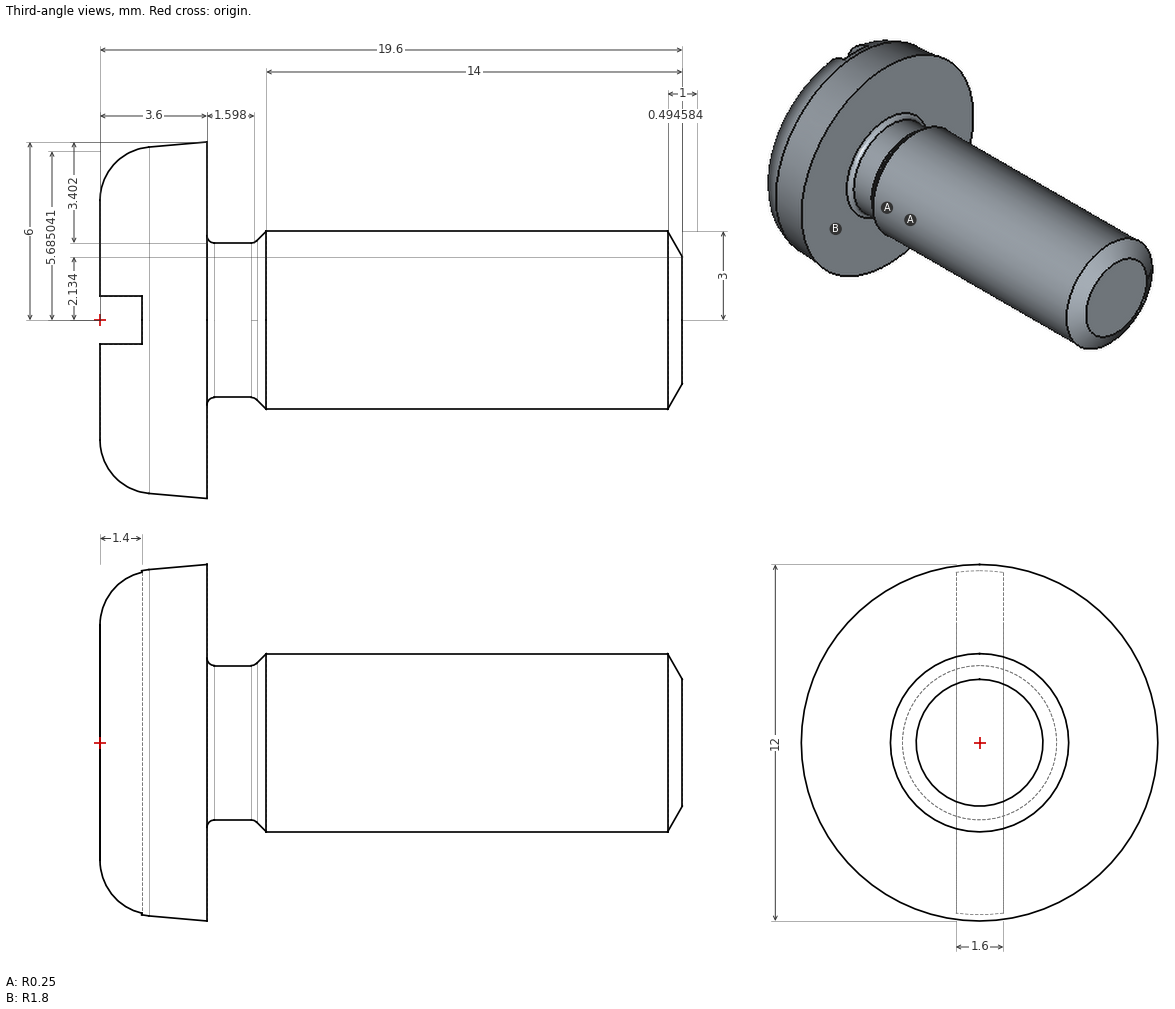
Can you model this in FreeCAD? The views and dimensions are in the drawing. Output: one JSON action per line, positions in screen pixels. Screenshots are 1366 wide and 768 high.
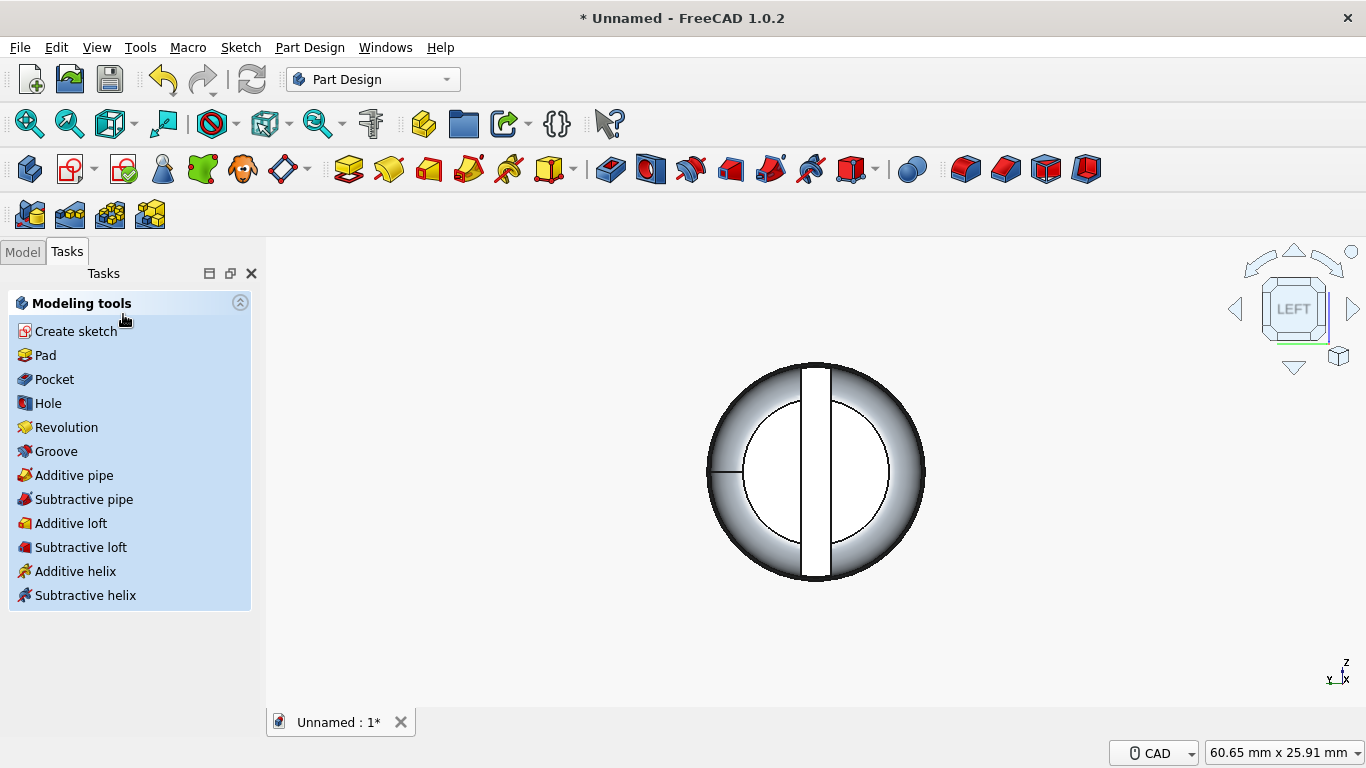
{"action": "left_click", "coordinate": [692, 170]}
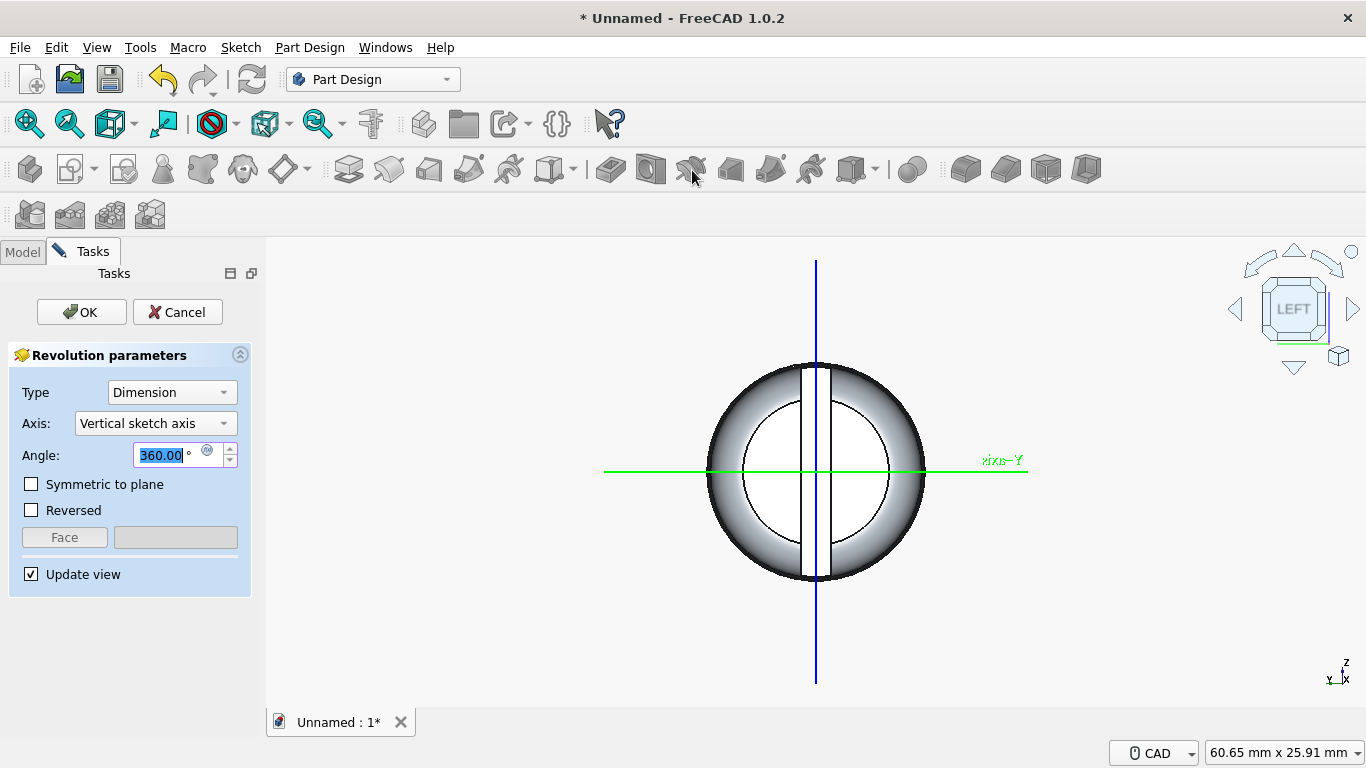
{"action": "left_click", "coordinate": [156, 424]}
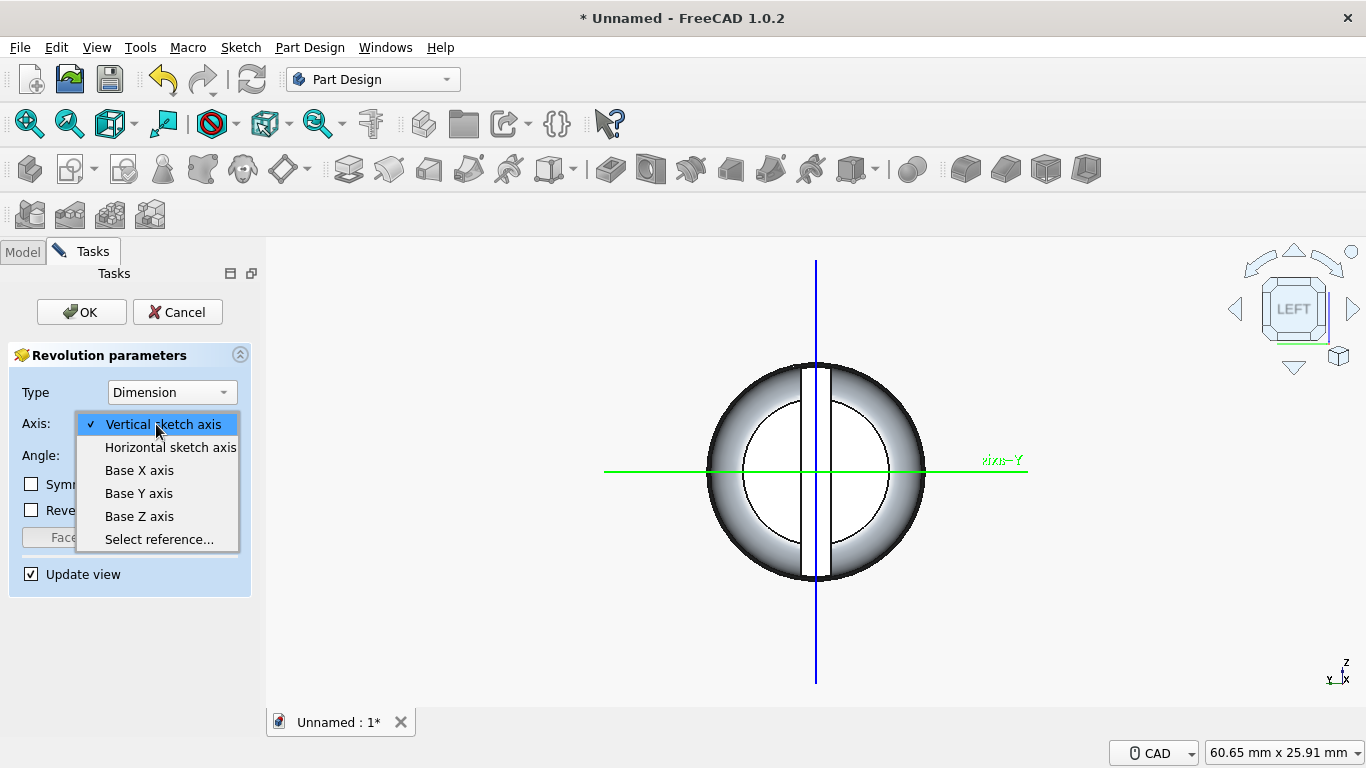
{"action": "left_click", "coordinate": [156, 448]}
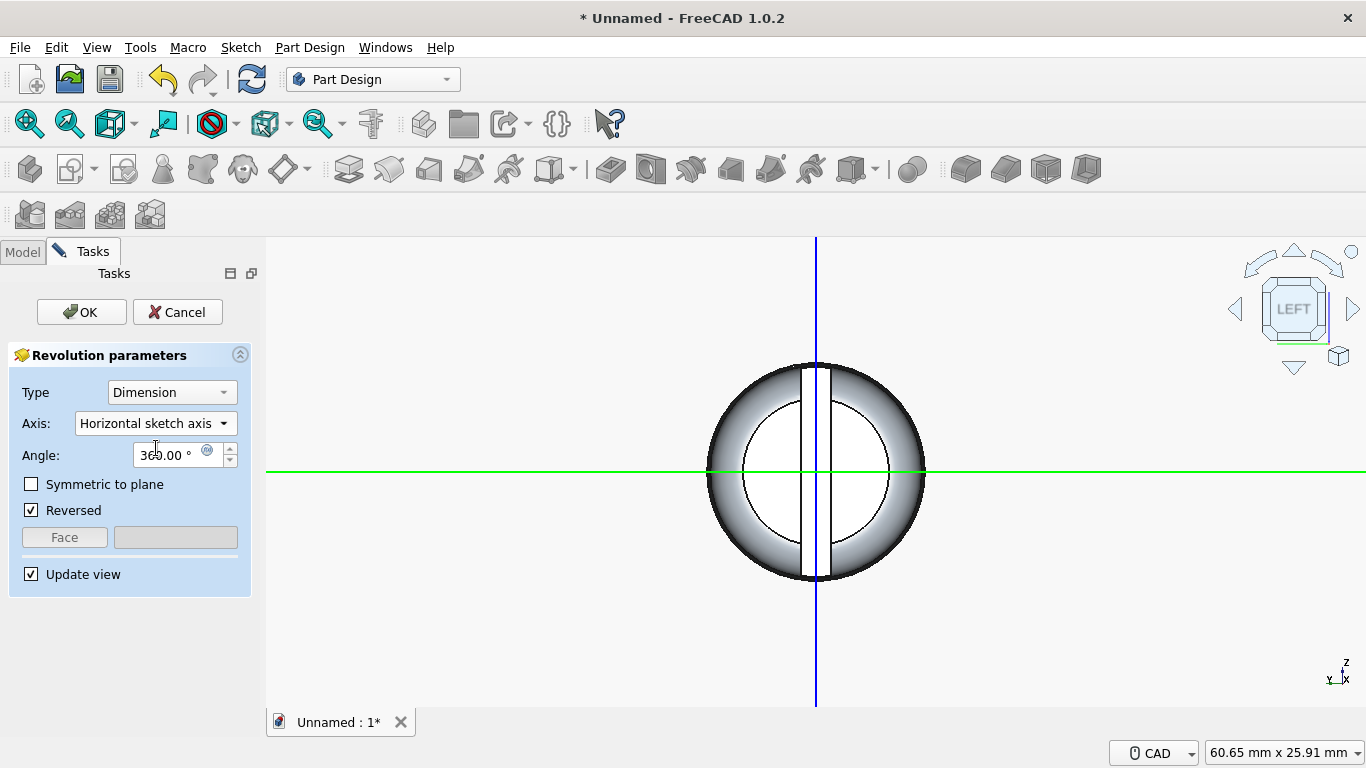
{"action": "left_click", "coordinate": [82, 312]}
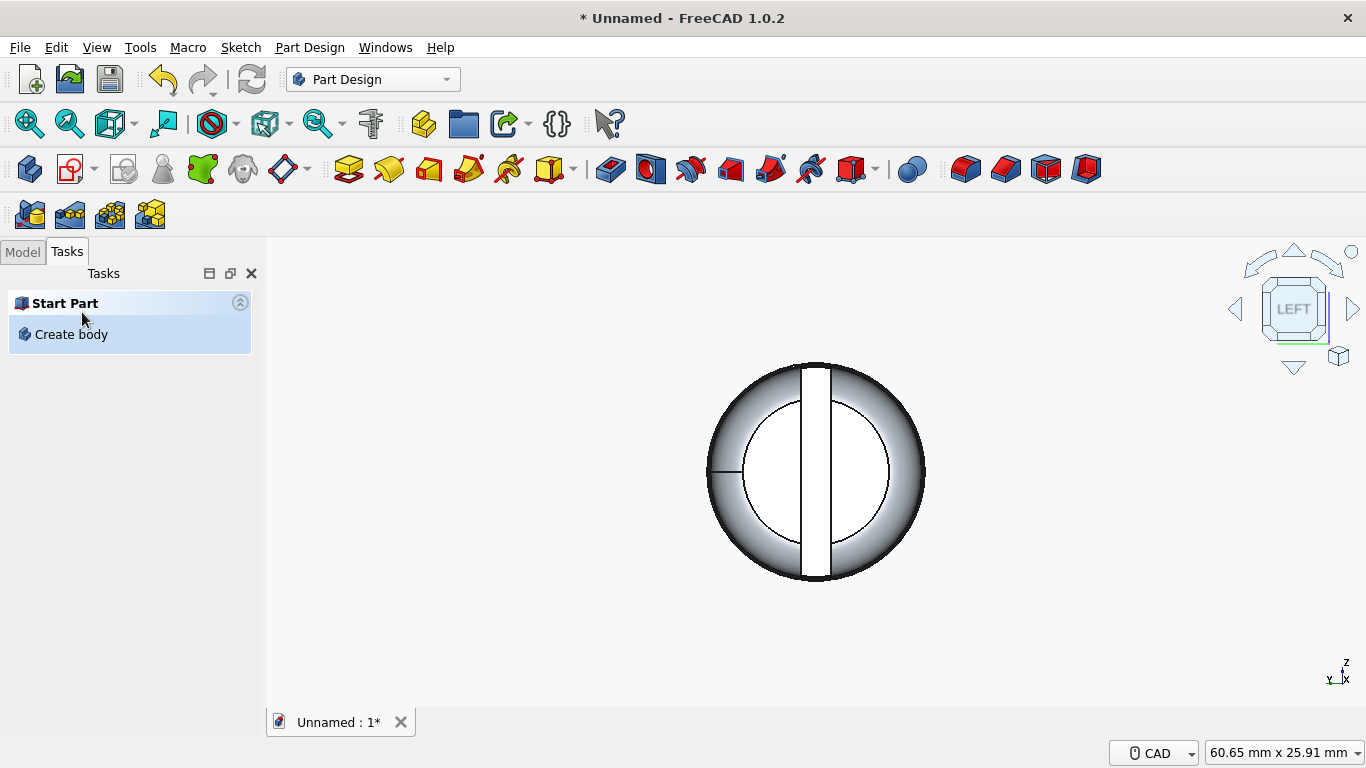
{"action": "key", "text": "0"}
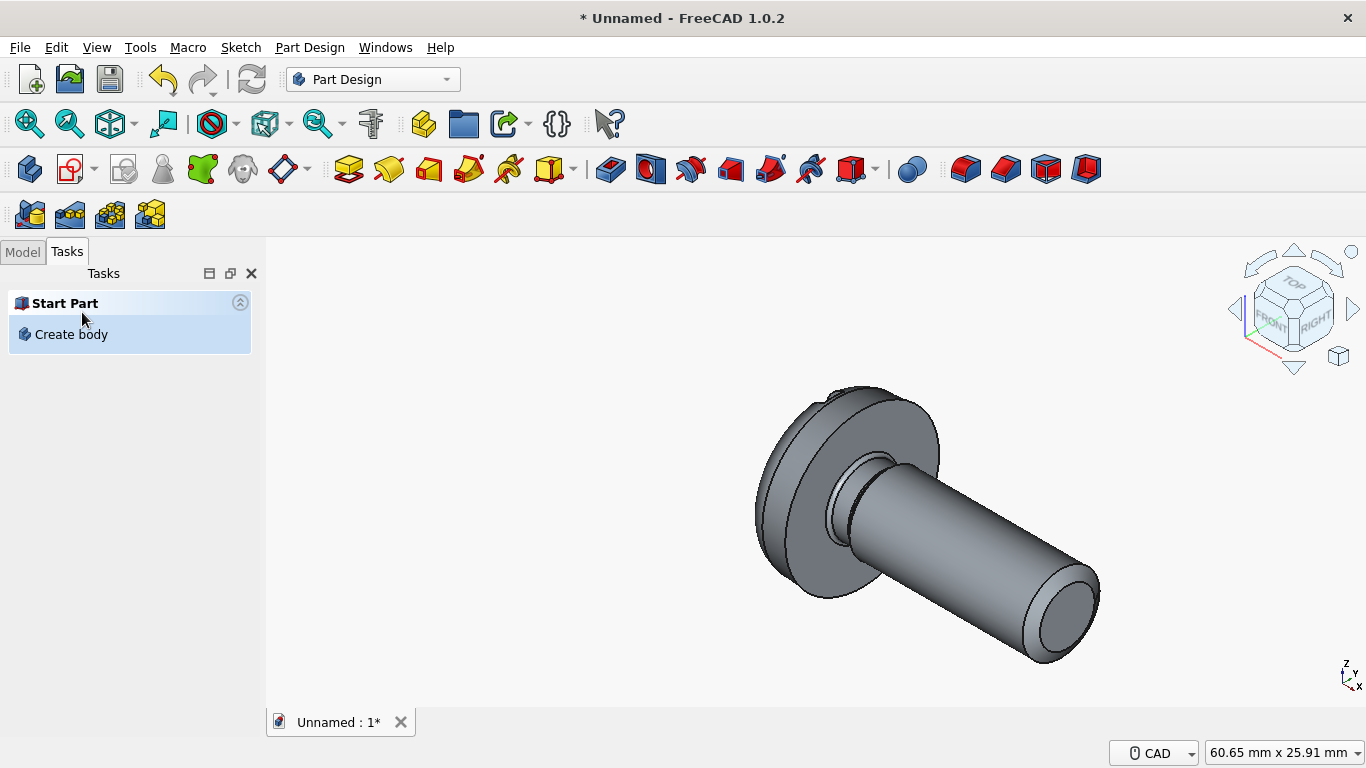
{"action": "left_click", "coordinate": [30, 124]}